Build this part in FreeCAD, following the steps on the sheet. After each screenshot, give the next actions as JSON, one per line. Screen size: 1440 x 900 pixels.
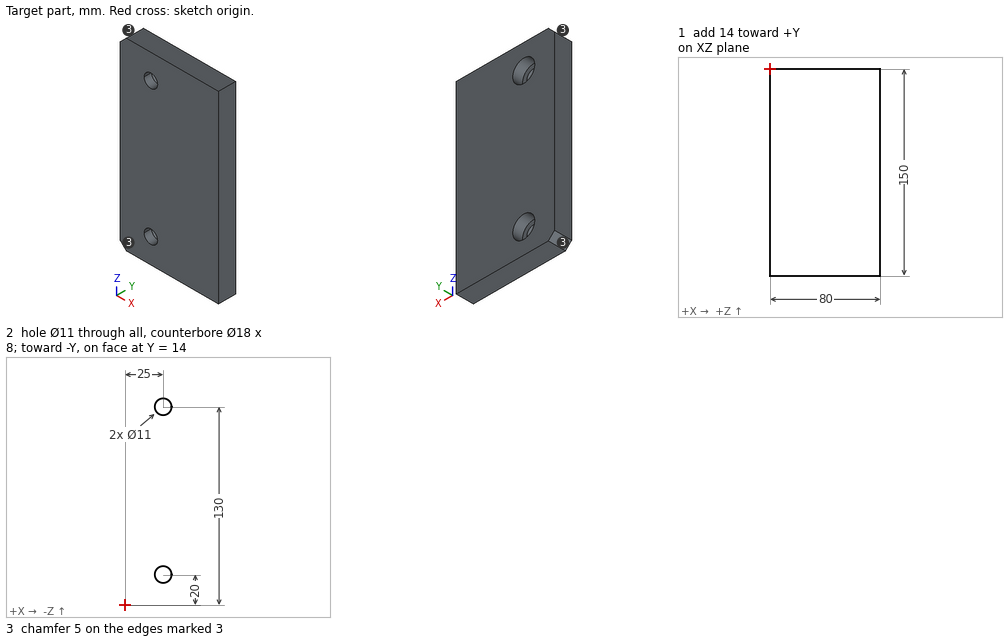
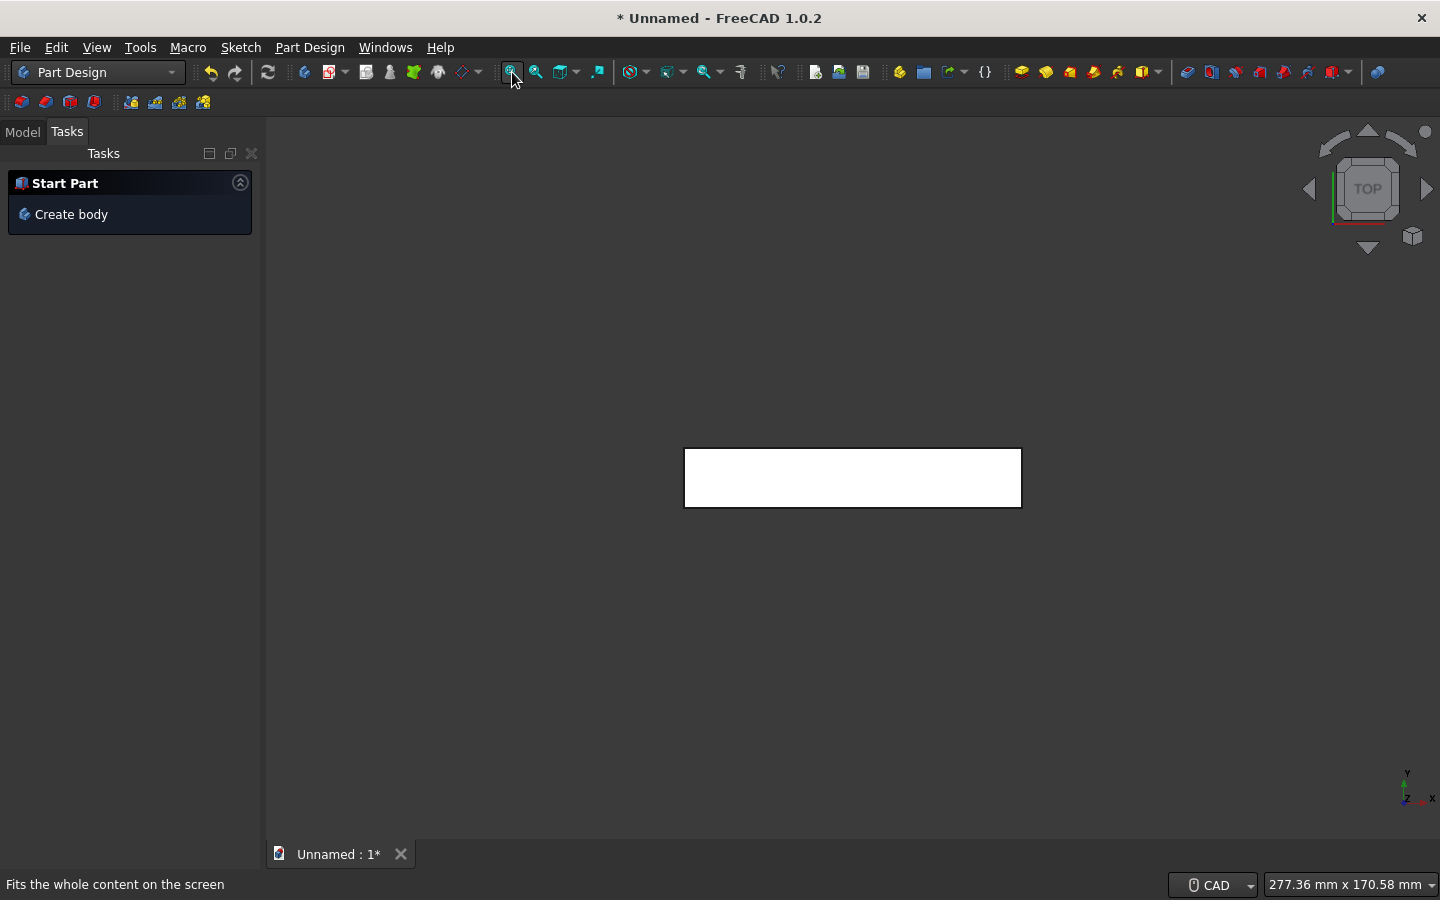
{"action": "left_click", "coordinate": [684, 477]}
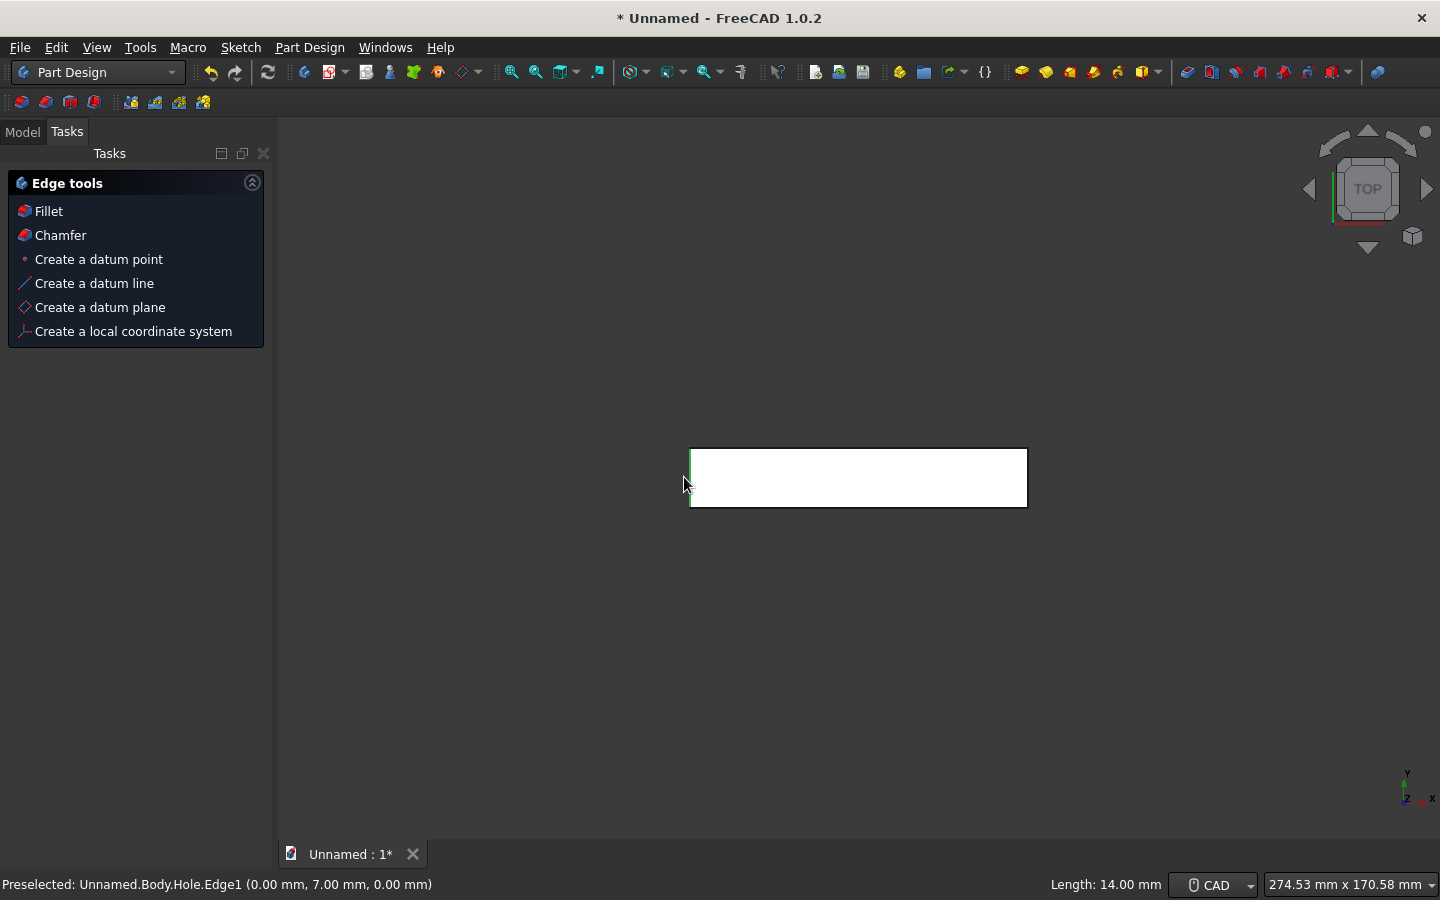
{"action": "key", "text": "1"}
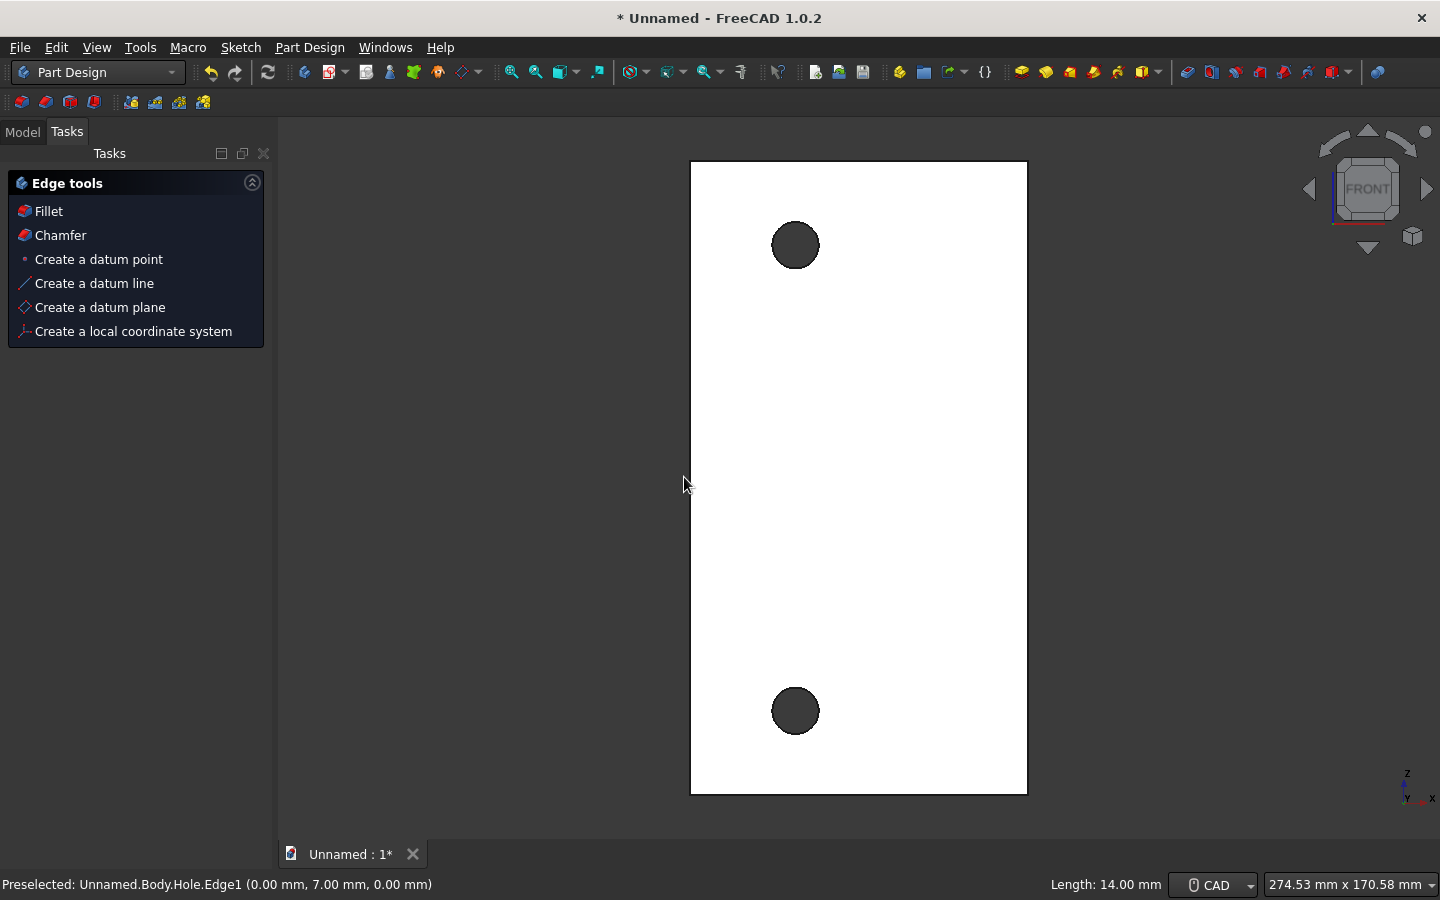
{"action": "key", "text": "3"}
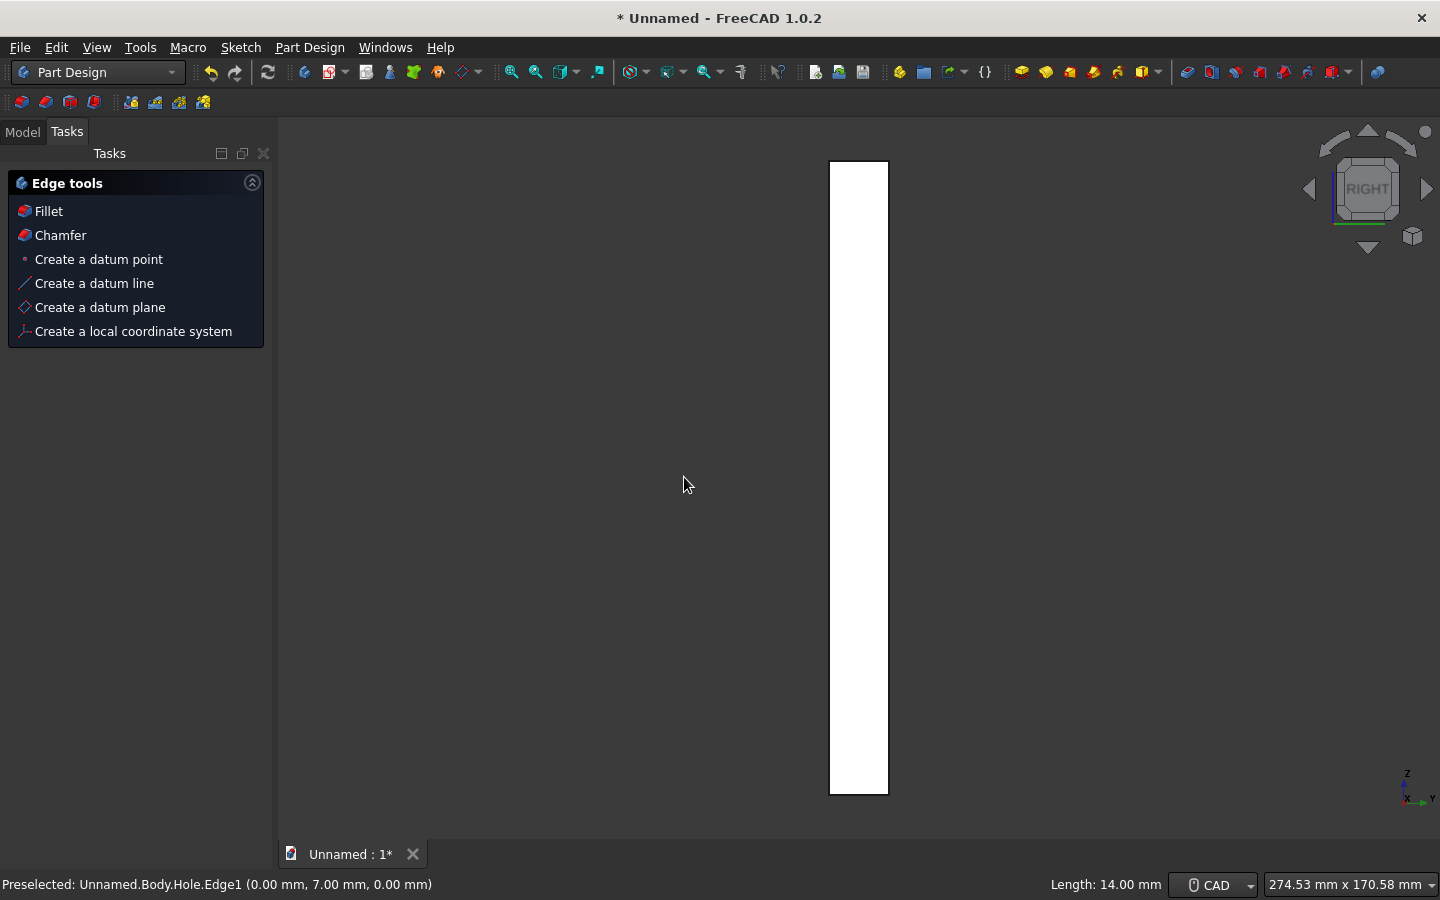
{"action": "key", "text": "5"}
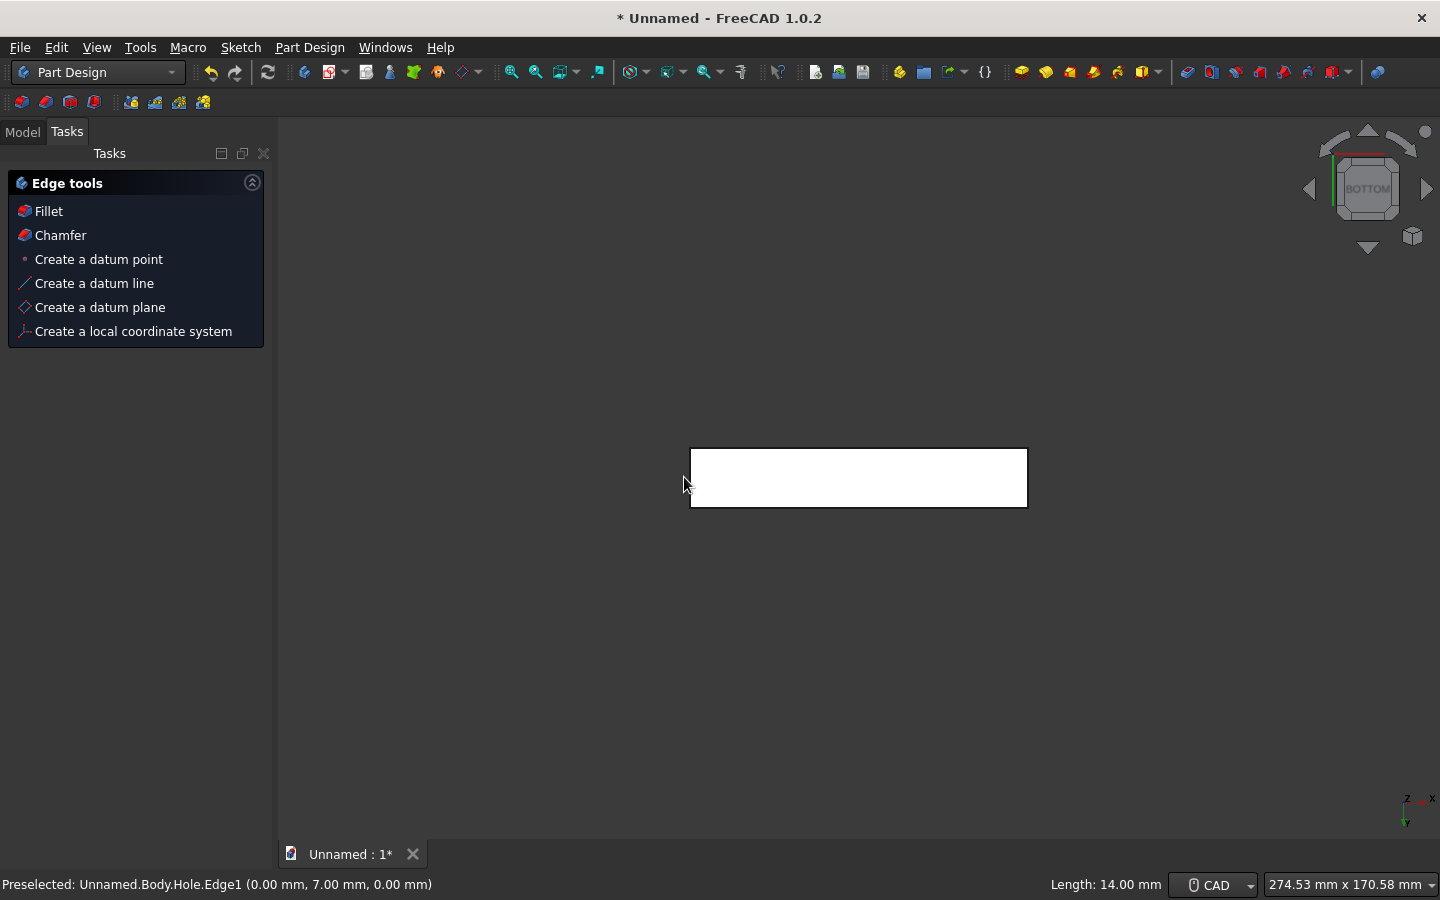
{"action": "left_click", "coordinate": [512, 72]}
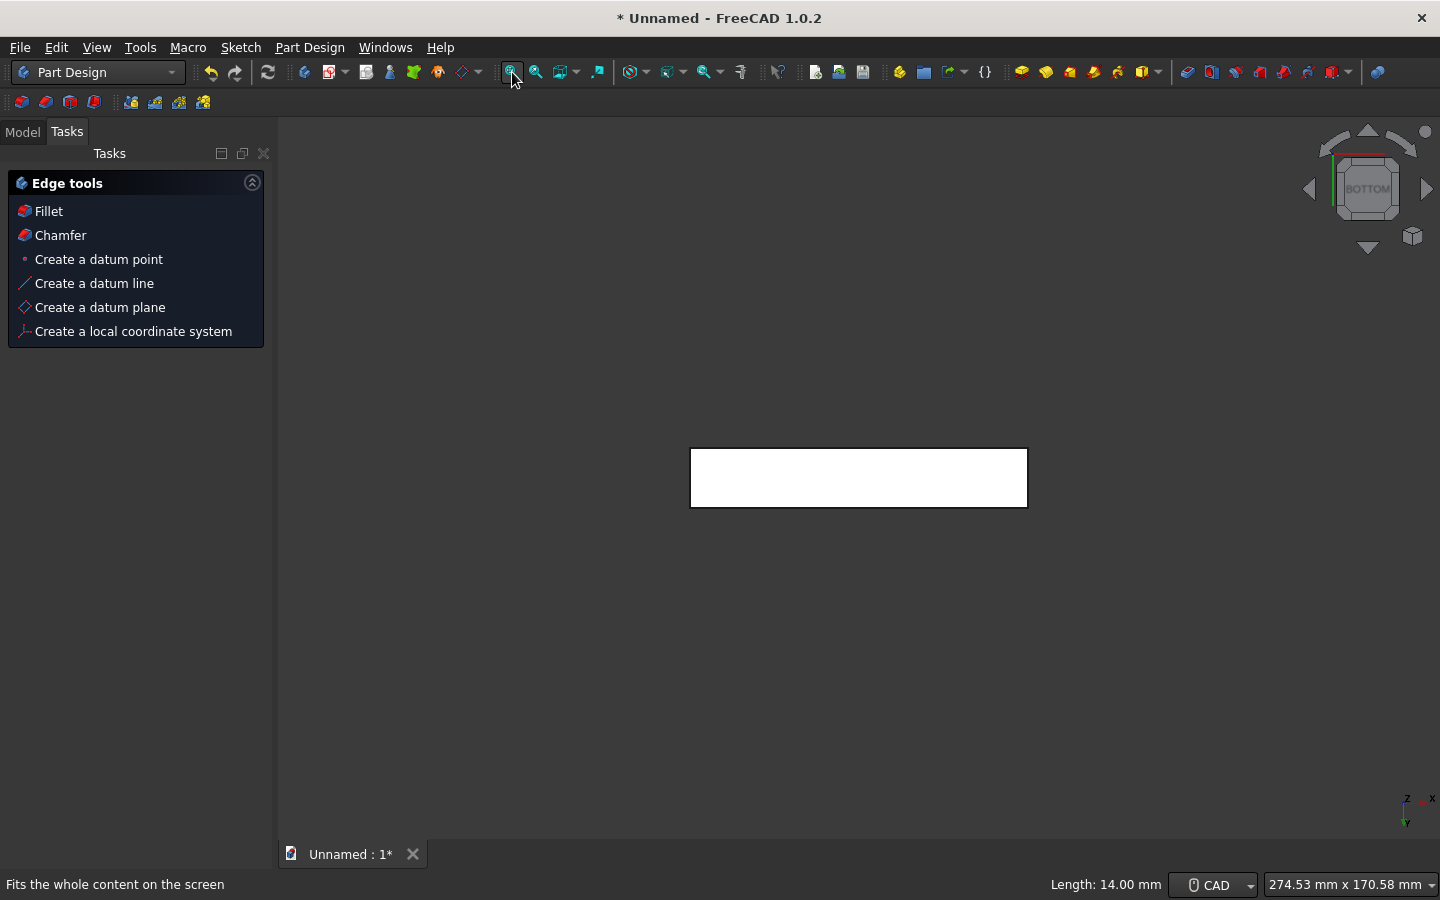
{"action": "left_click", "coordinate": [690, 477], "text": "ctrl"}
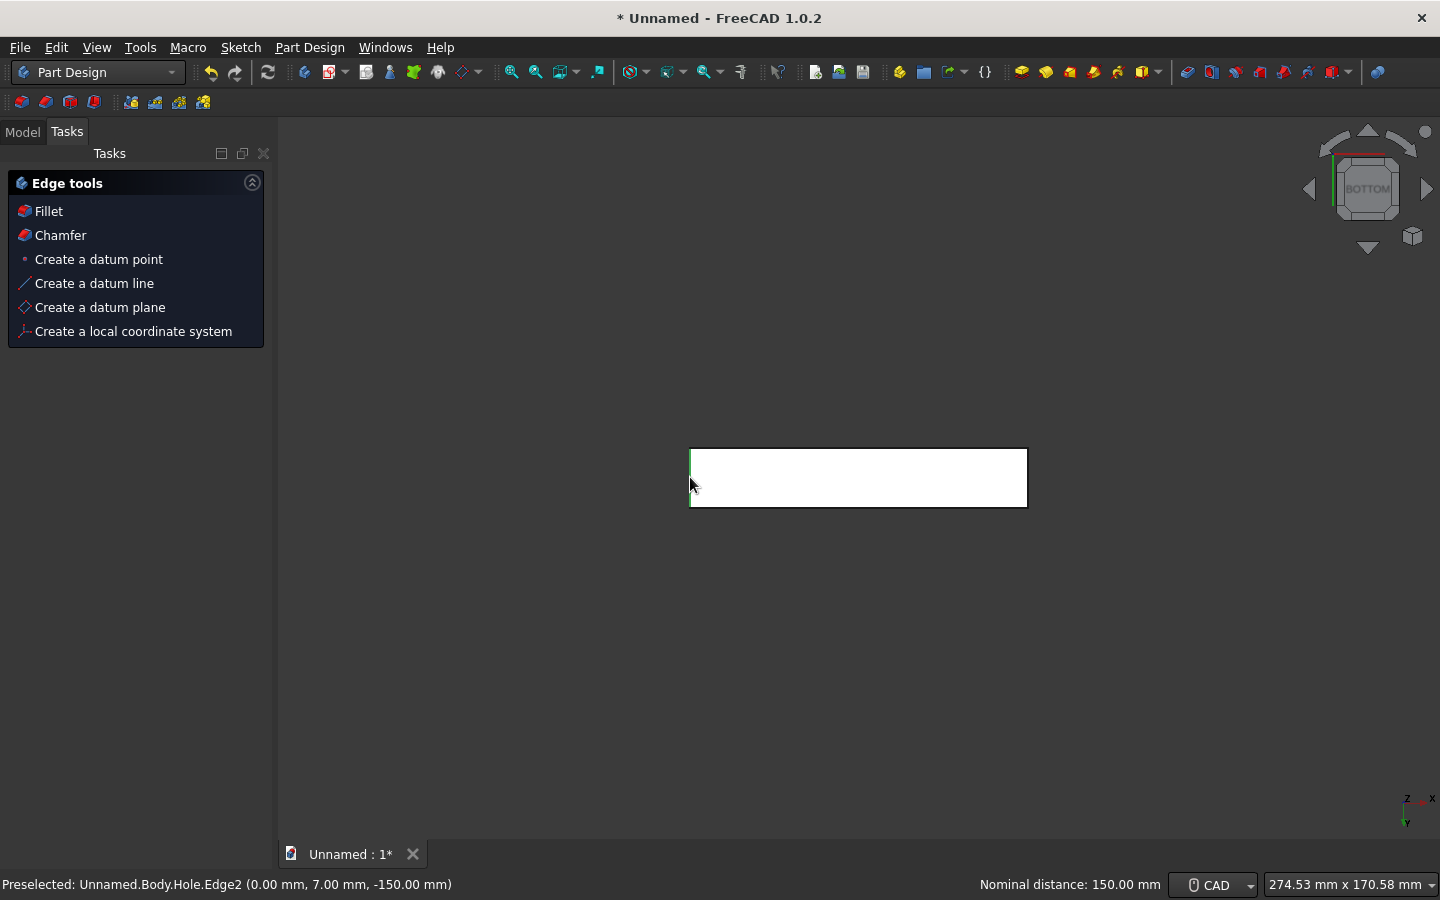
{"action": "left_click", "coordinate": [46, 102]}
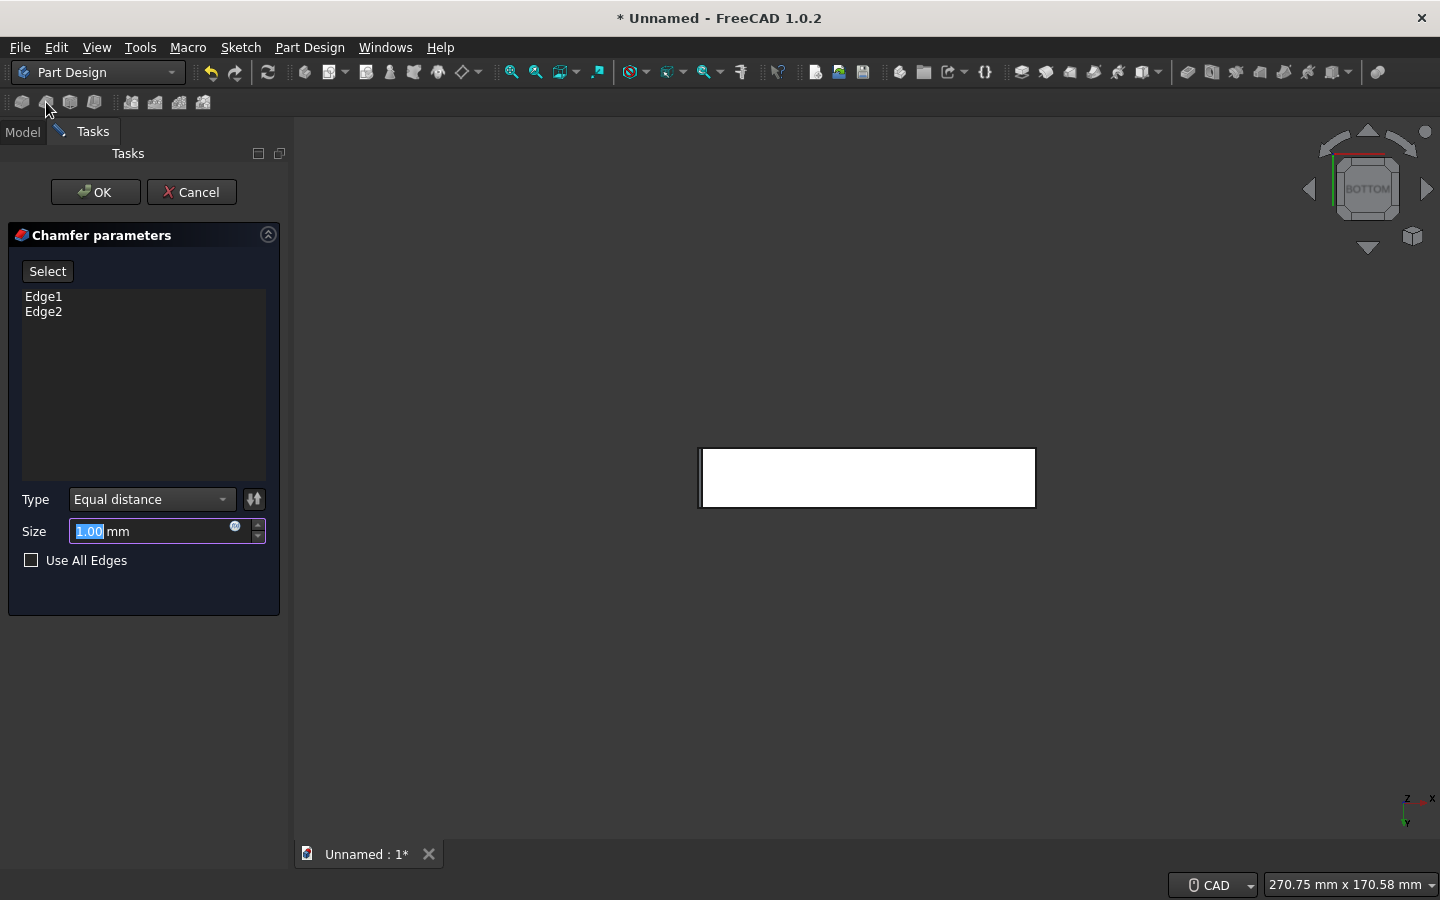
{"action": "type", "text": "5"}
{"action": "key", "text": "Tab"}